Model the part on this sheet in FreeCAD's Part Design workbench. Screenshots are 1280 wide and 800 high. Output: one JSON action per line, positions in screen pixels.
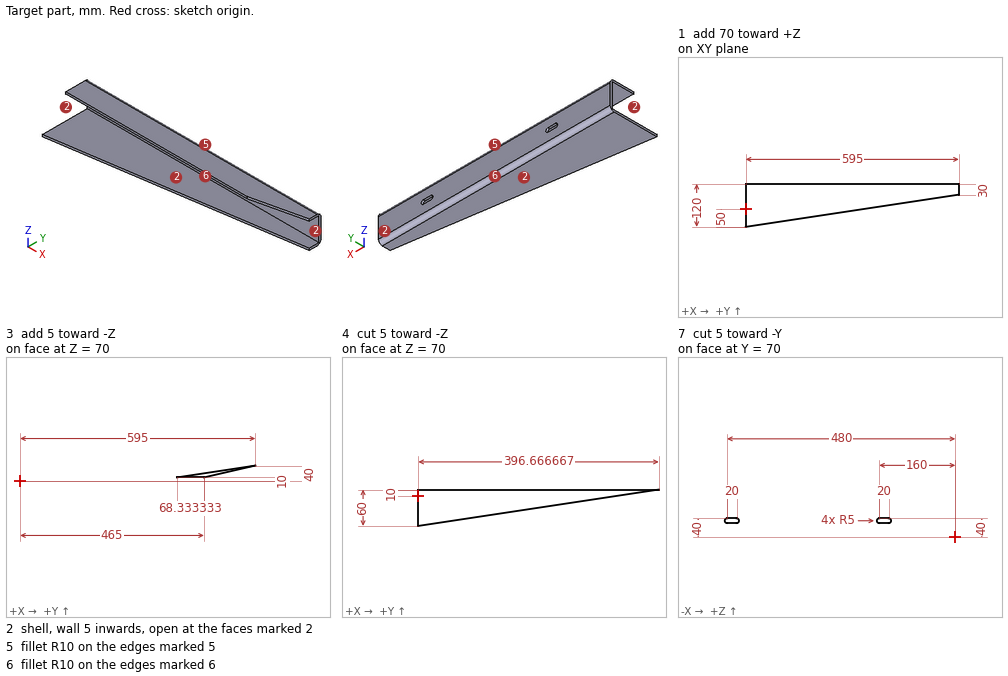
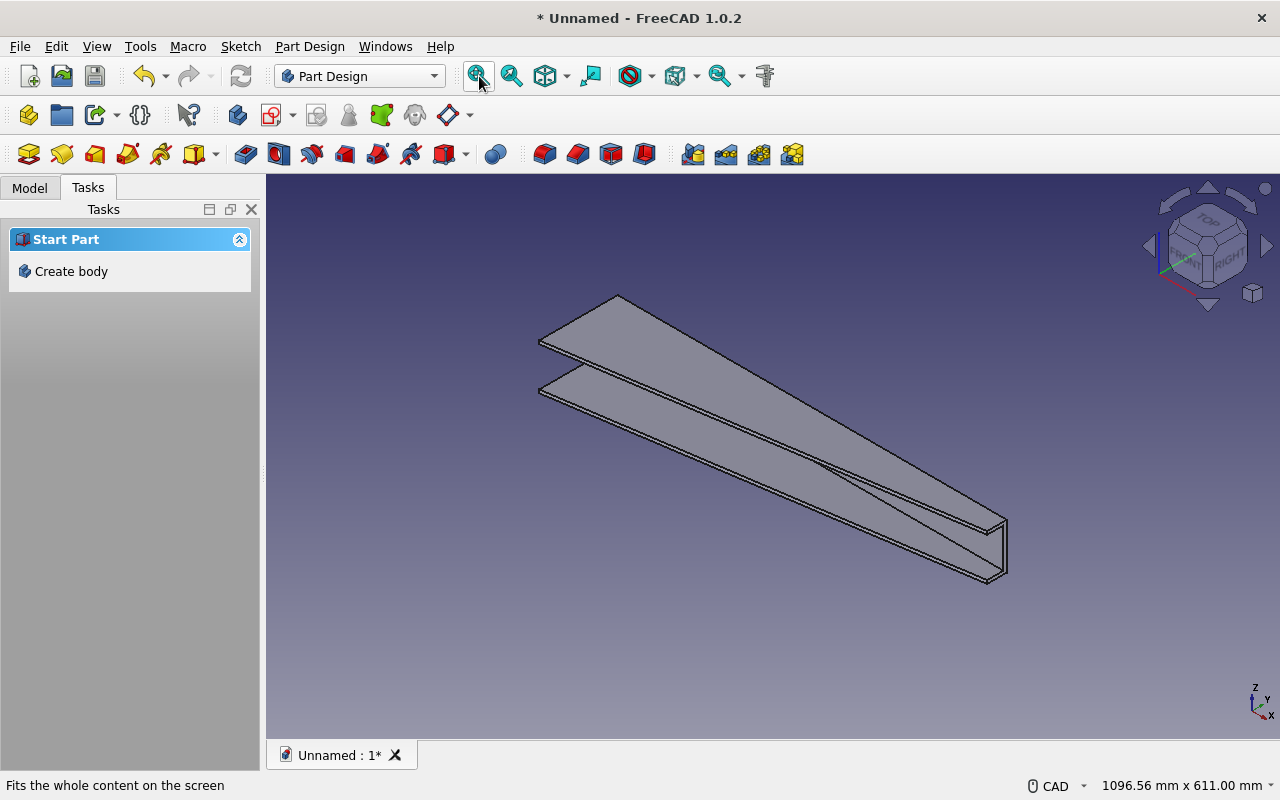
{"action": "left_click", "coordinate": [729, 391]}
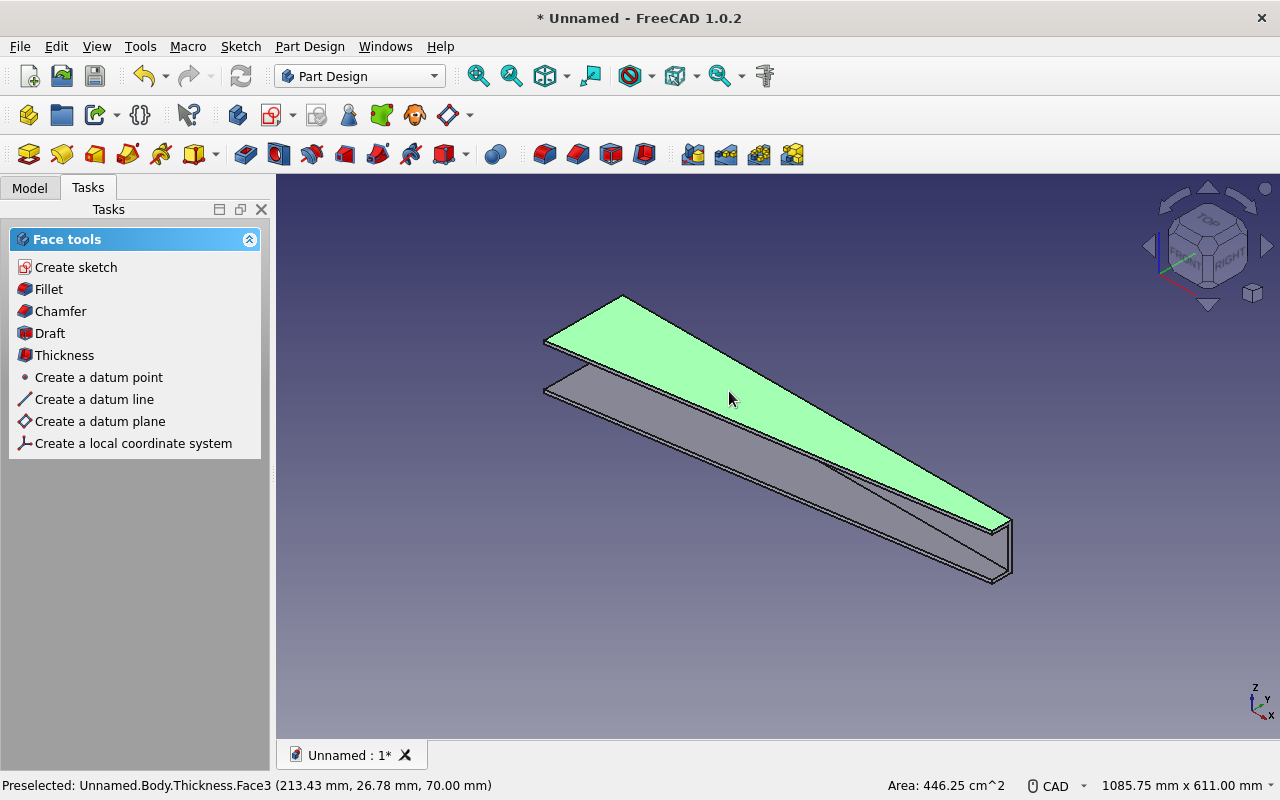
{"action": "left_click", "coordinate": [270, 116]}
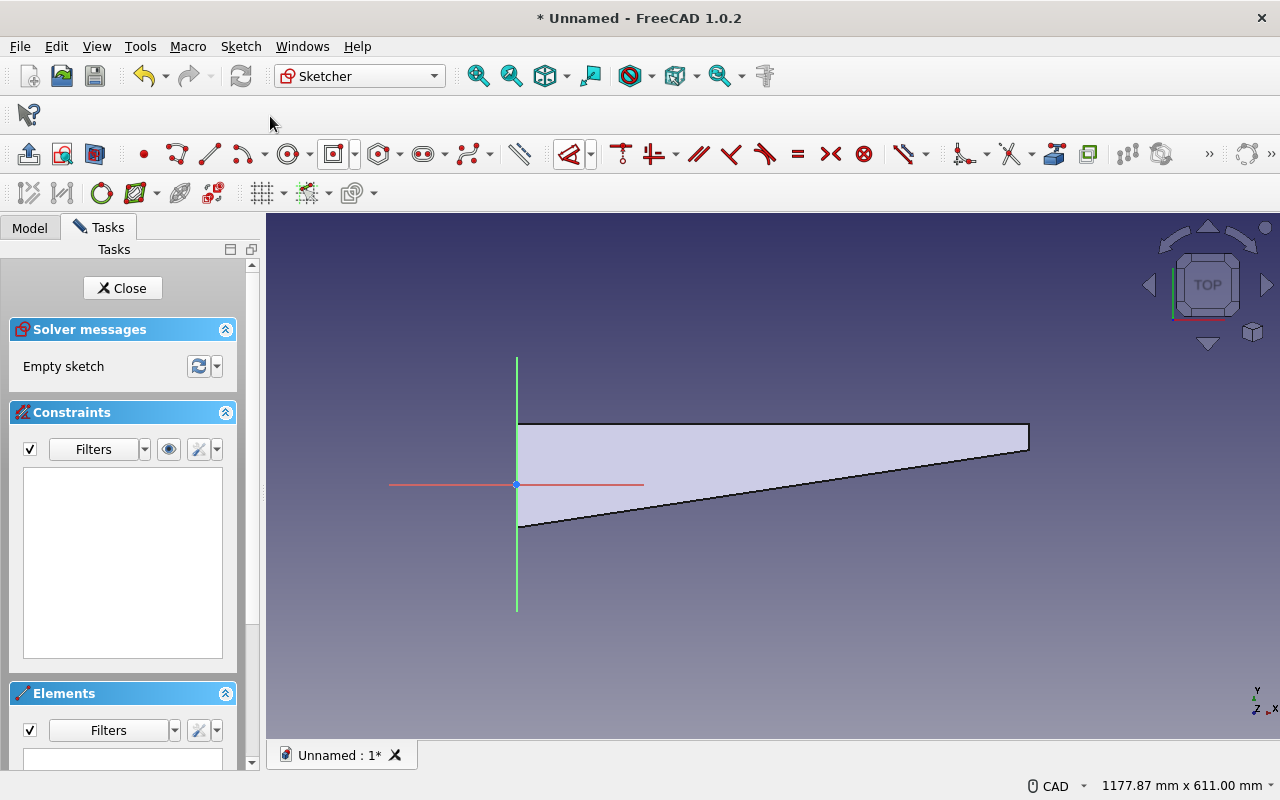
{"action": "scroll", "coordinate": [1047, 458], "scroll_direction": "up", "scroll_amount": 6}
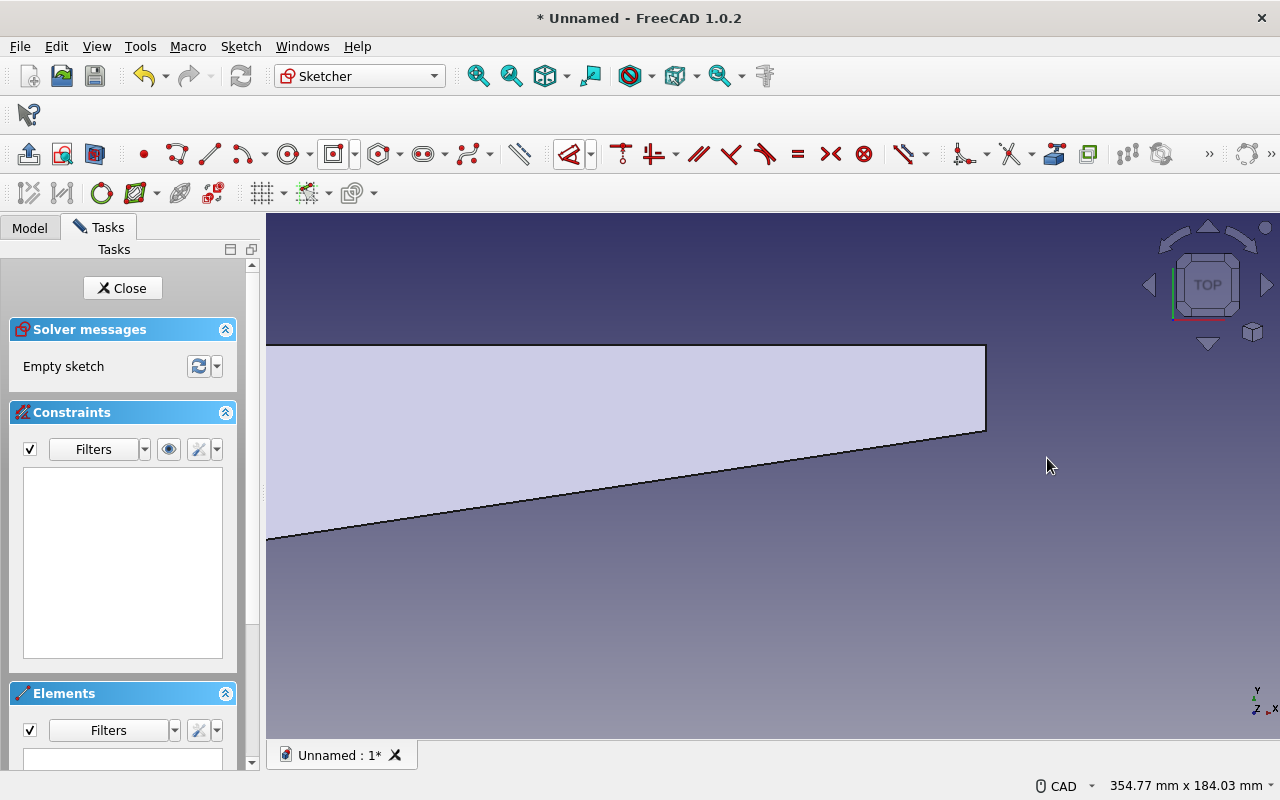
{"action": "left_click", "coordinate": [177, 154]}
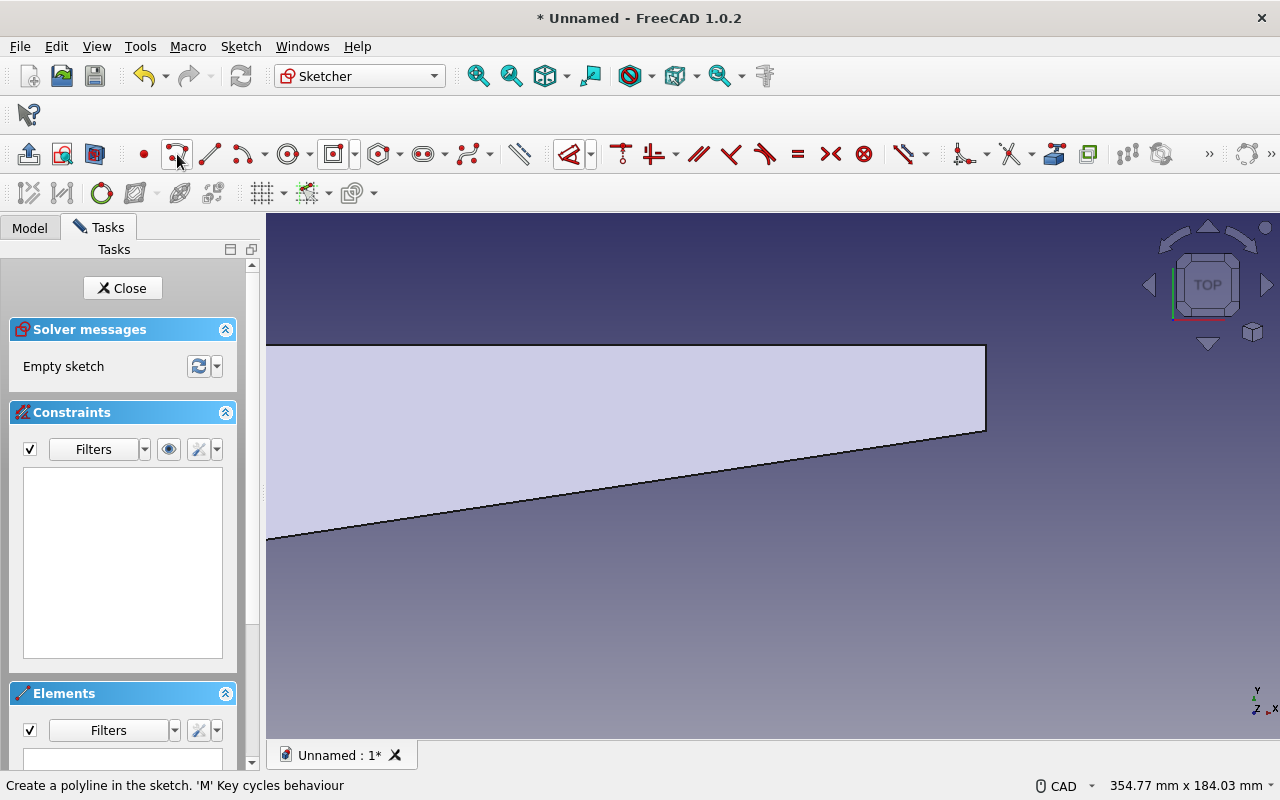
{"action": "left_click", "coordinate": [419, 517]}
{"action": "left_click", "coordinate": [614, 517]}
{"action": "left_click", "coordinate": [986, 431]}
{"action": "left_click", "coordinate": [419, 518]}
{"action": "key", "text": "Escape"}
{"action": "key", "text": "Escape"}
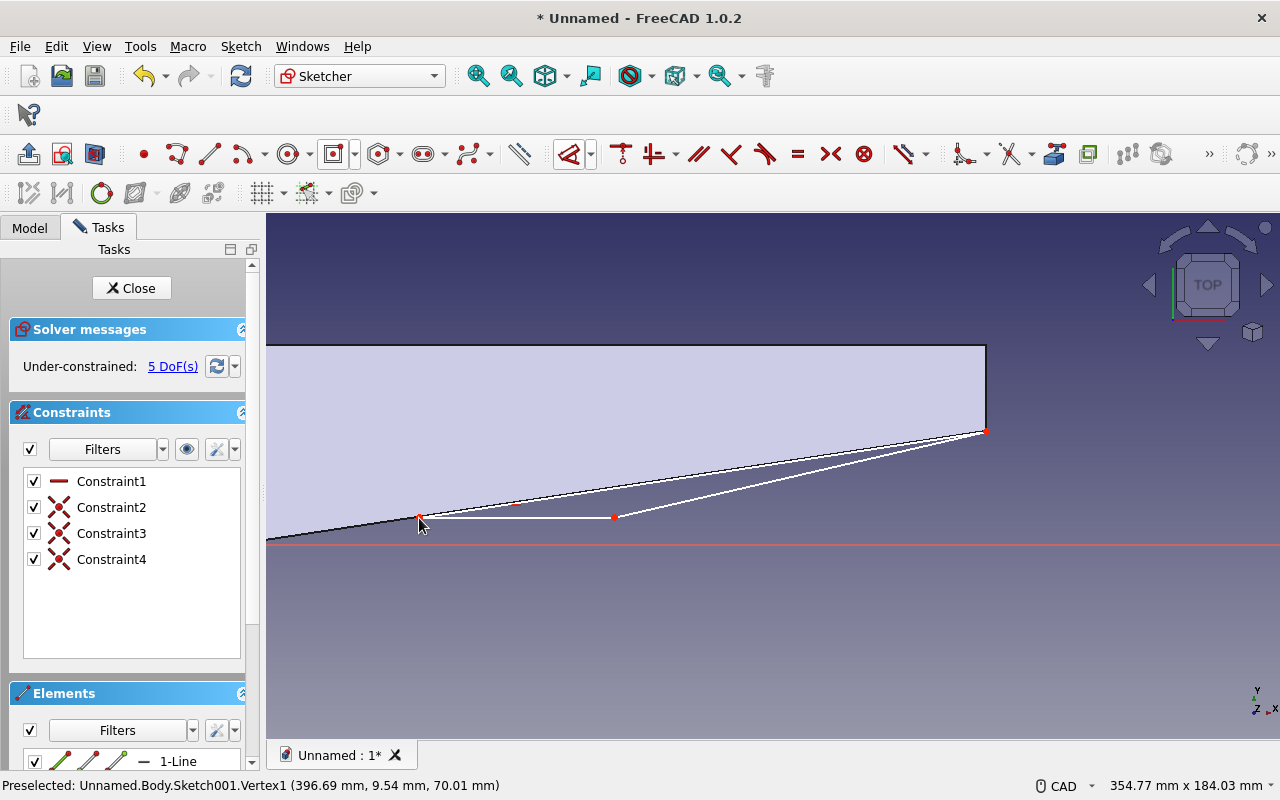
{"action": "scroll", "coordinate": [419, 518], "scroll_direction": "up", "scroll_amount": 2}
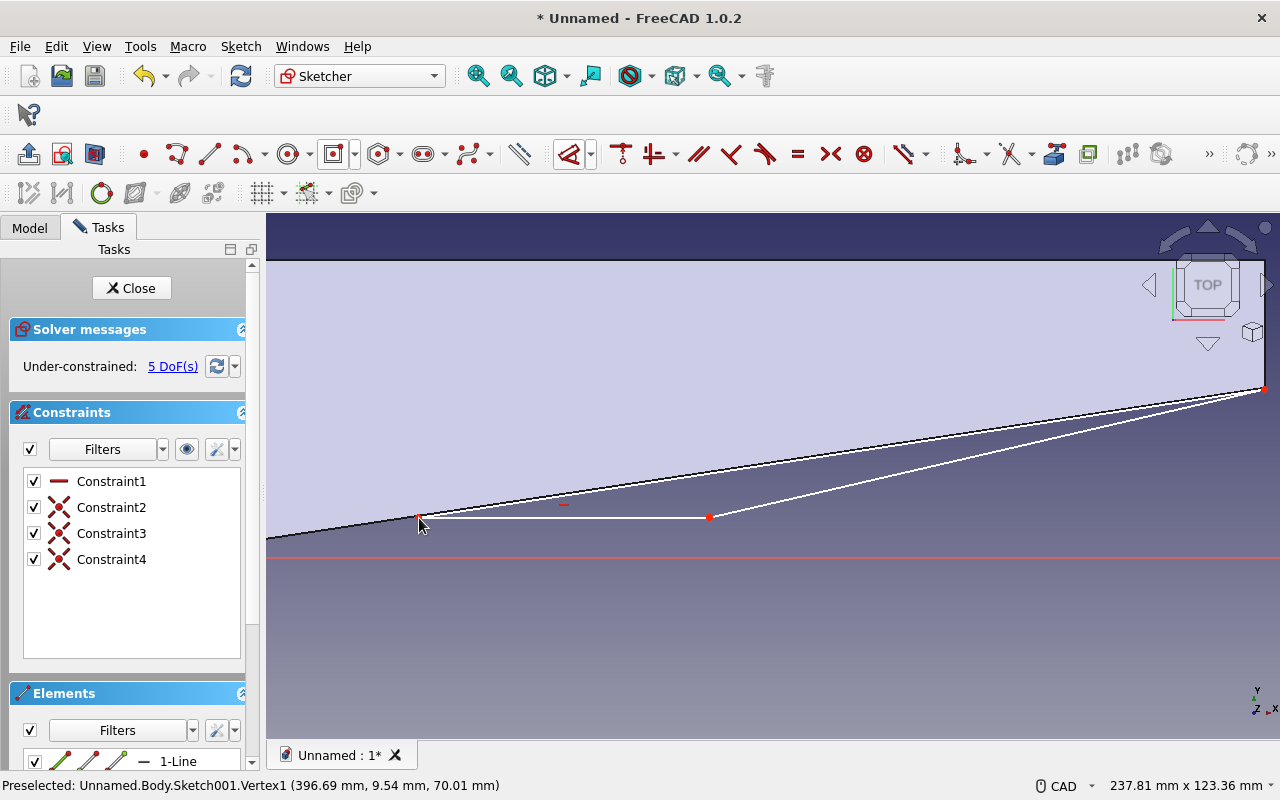
{"action": "left_click", "coordinate": [419, 518]}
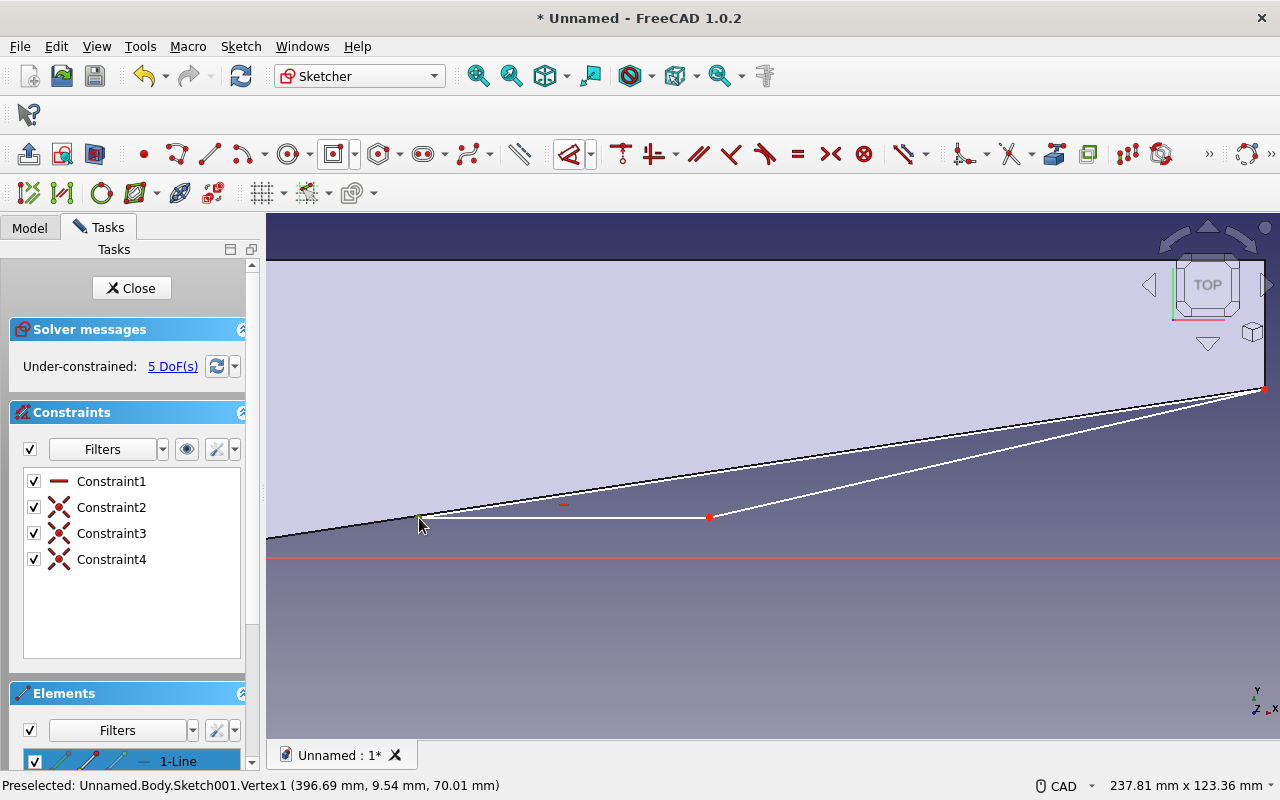
{"action": "key", "text": "i"}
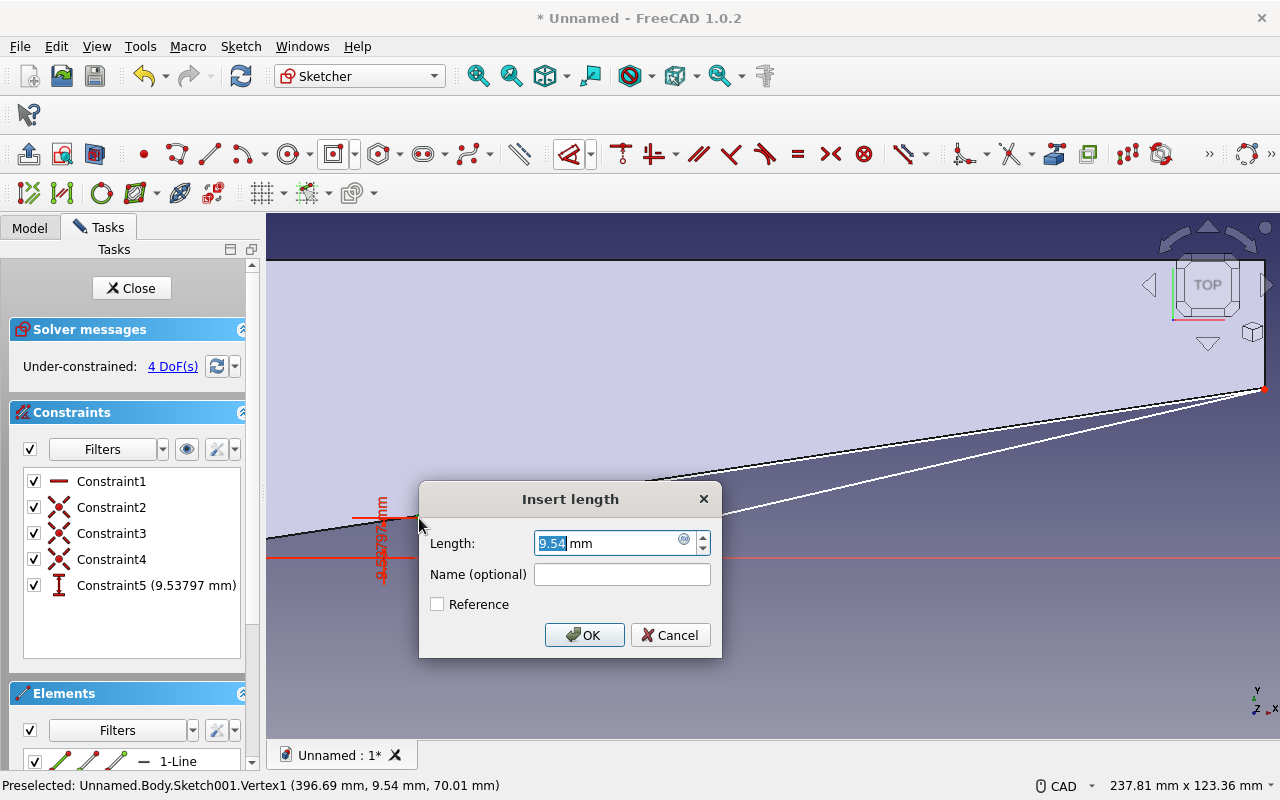
{"action": "type", "text": "10"}
{"action": "key", "text": "Return"}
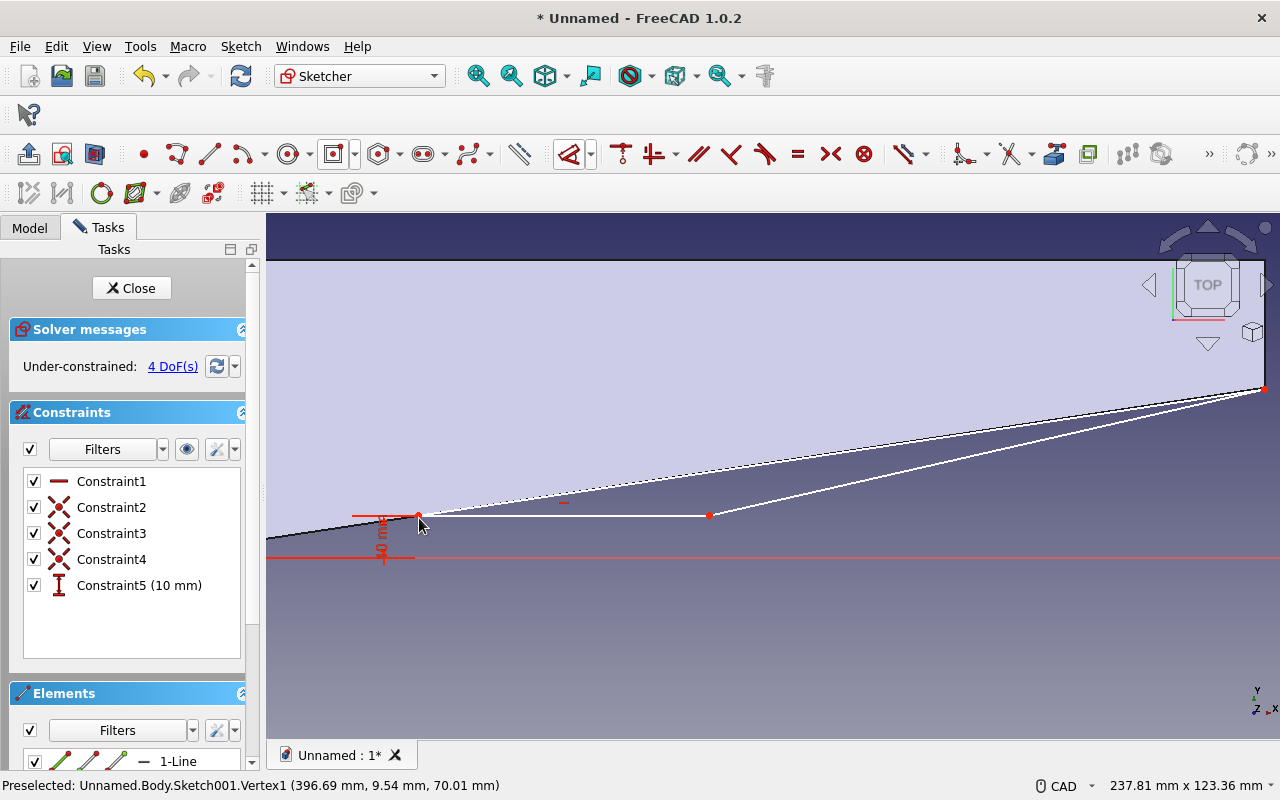
{"action": "scroll", "coordinate": [426, 525], "scroll_direction": "down", "scroll_amount": 2}